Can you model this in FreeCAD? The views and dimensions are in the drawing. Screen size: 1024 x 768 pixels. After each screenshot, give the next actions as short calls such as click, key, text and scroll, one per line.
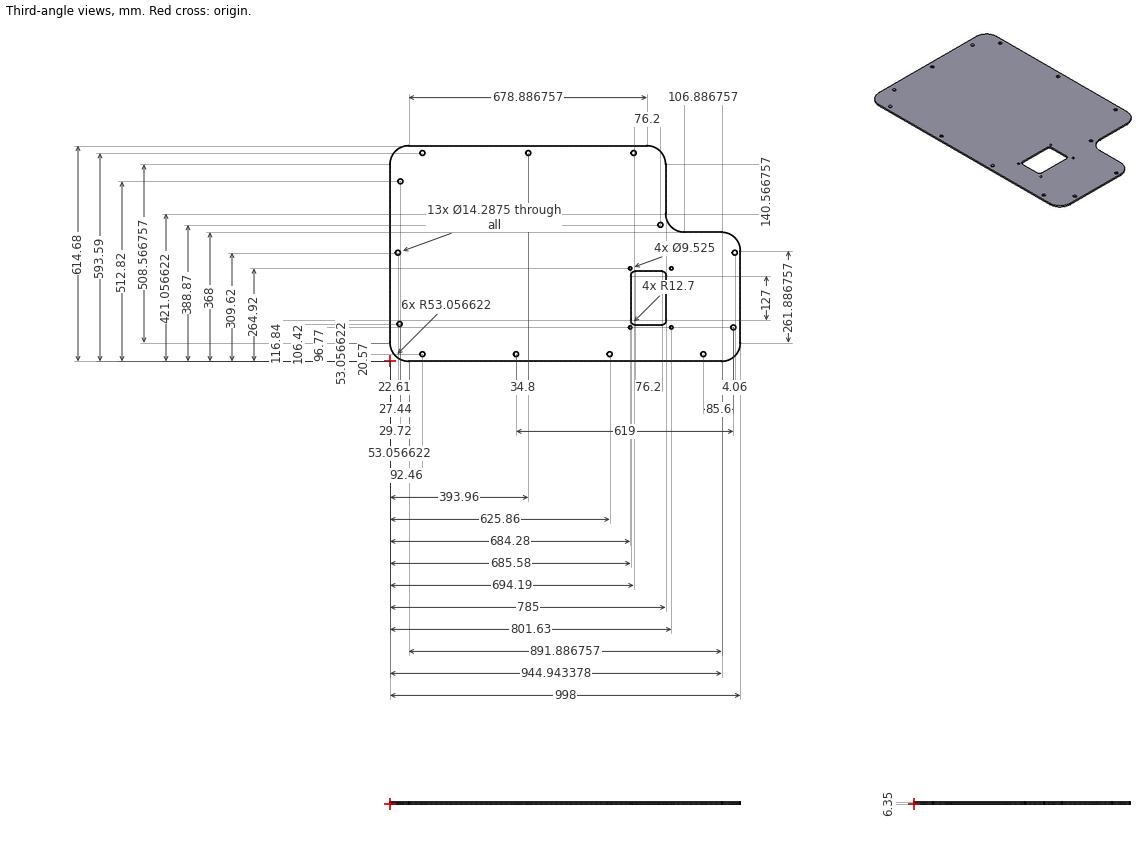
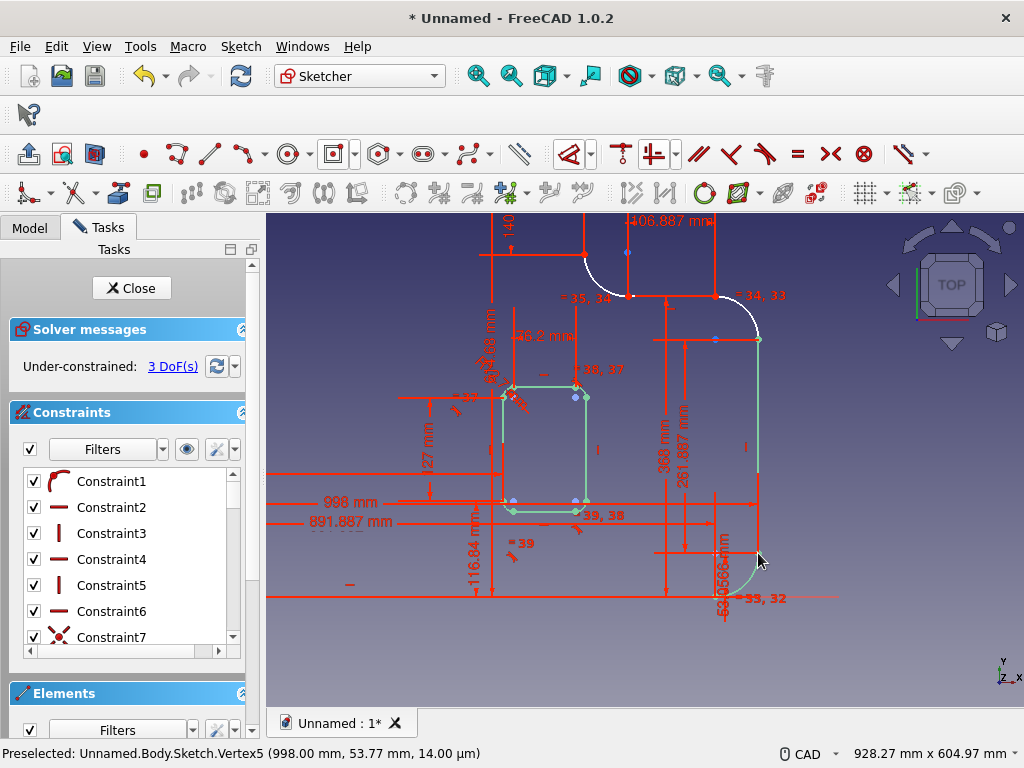
scroll(761, 553, down, 4)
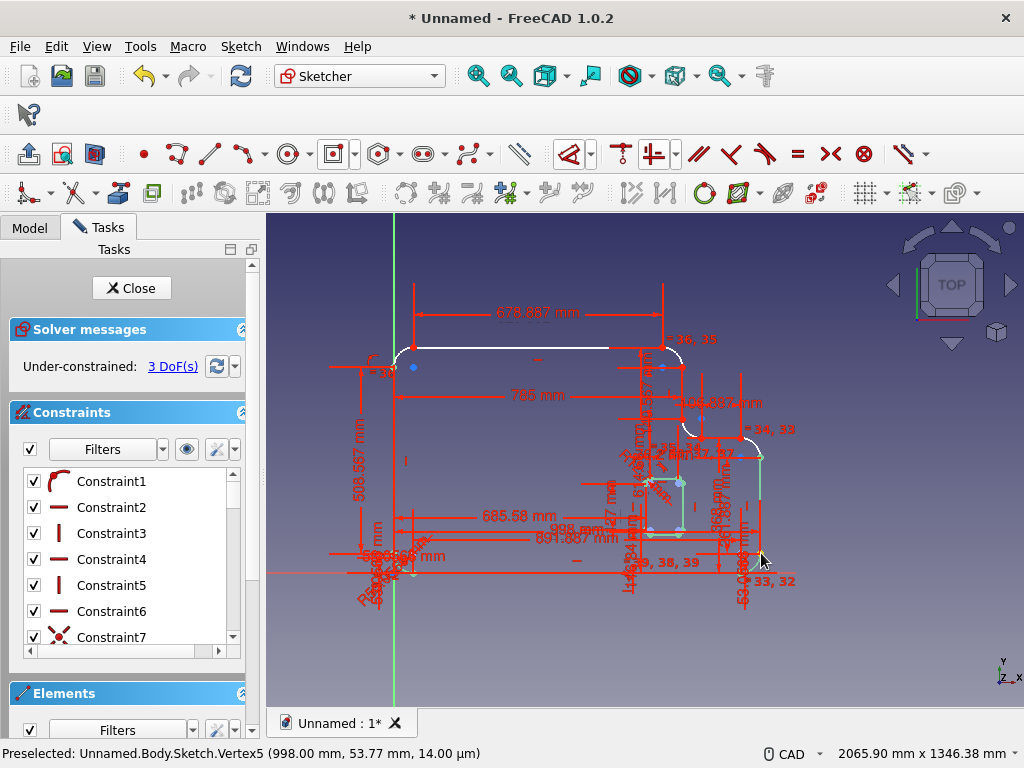
scroll(414, 348, up, 4)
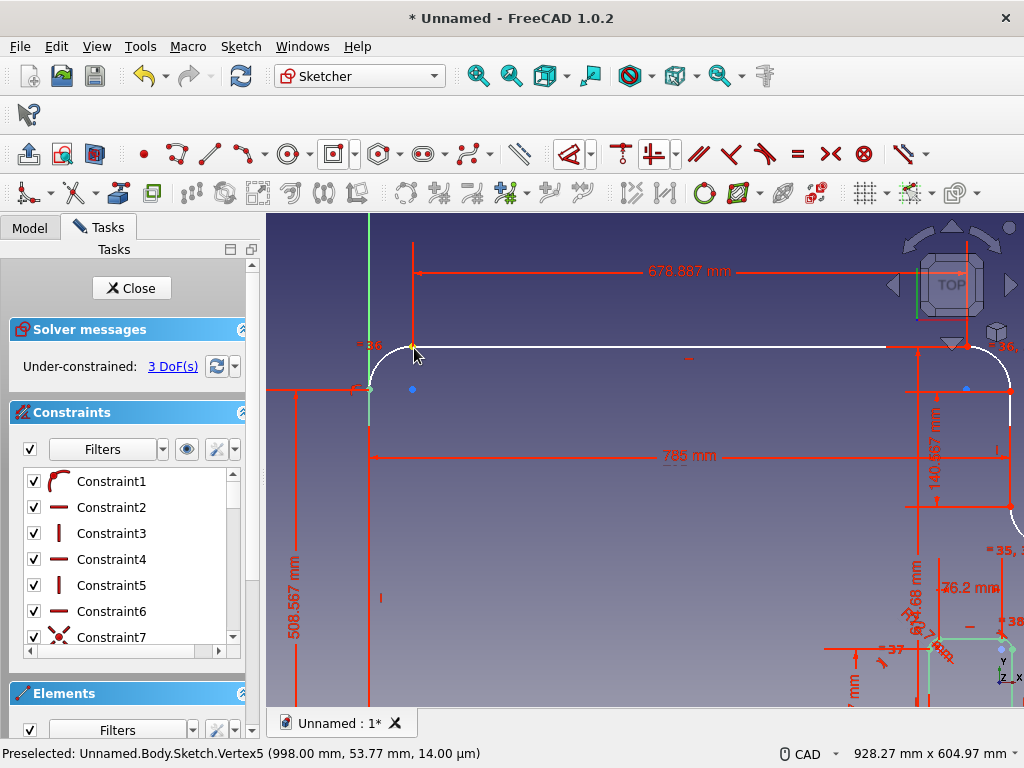
click(413, 347)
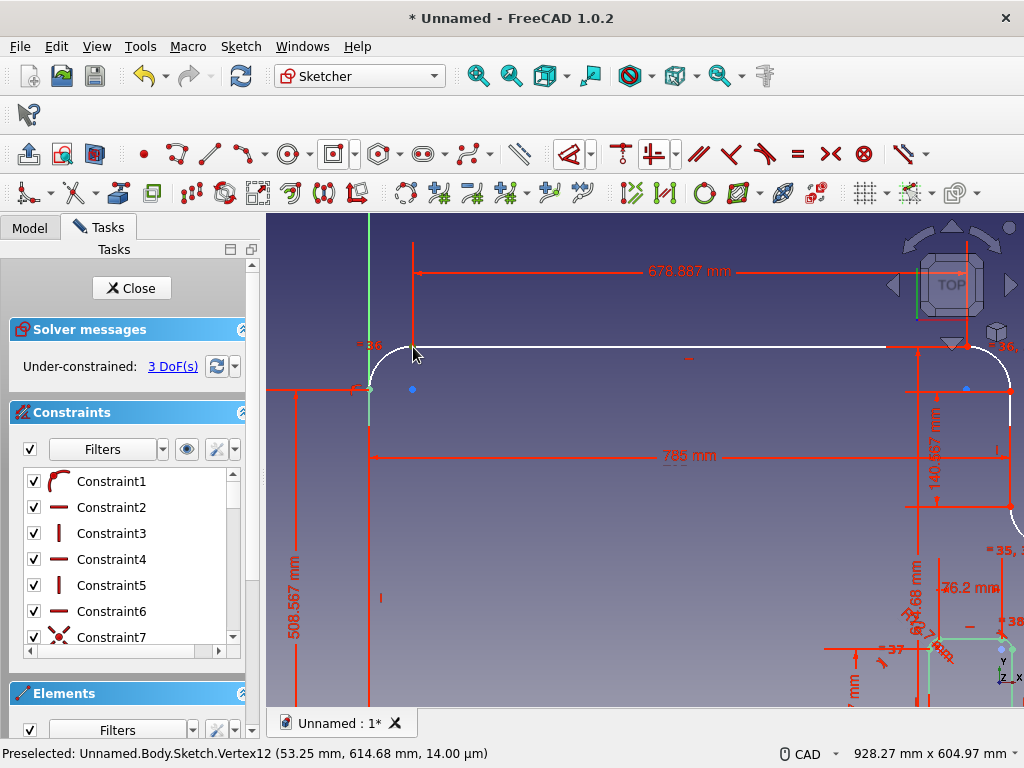
click(590, 154)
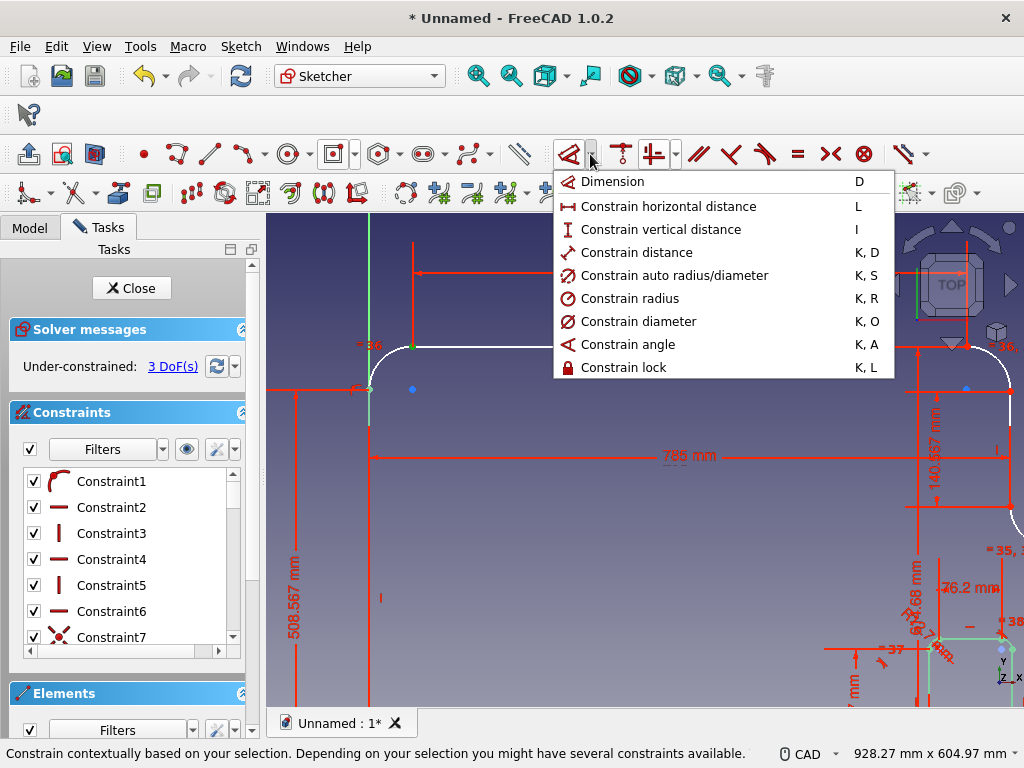
click(724, 206)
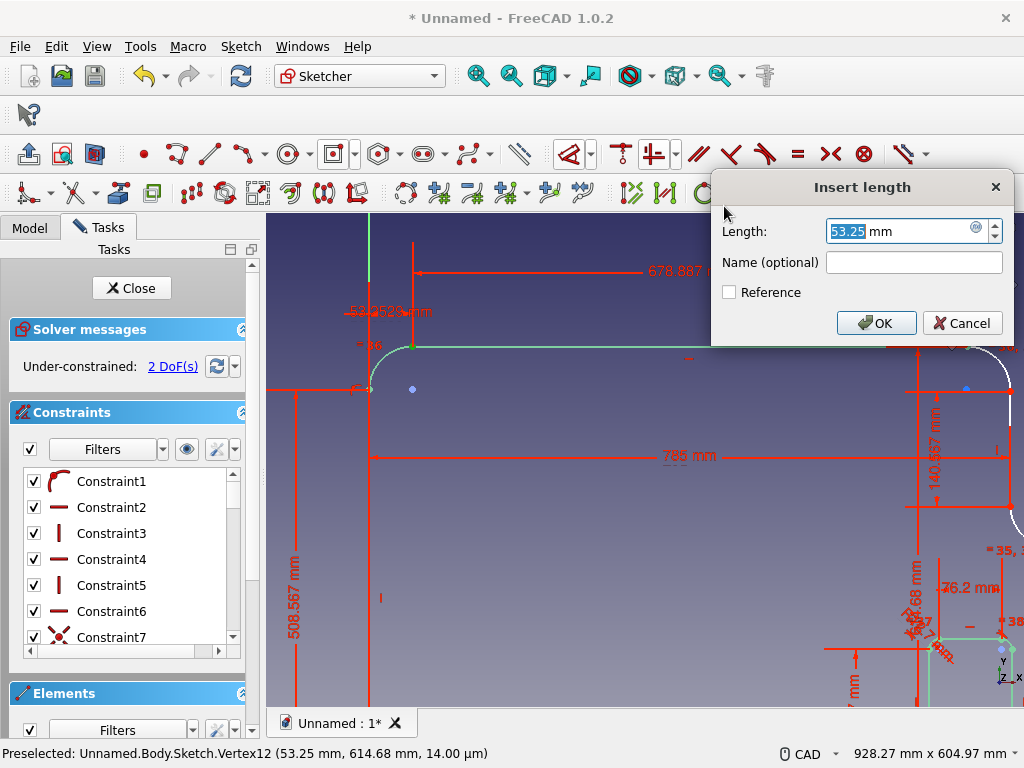
text(53.056622)
key(Return)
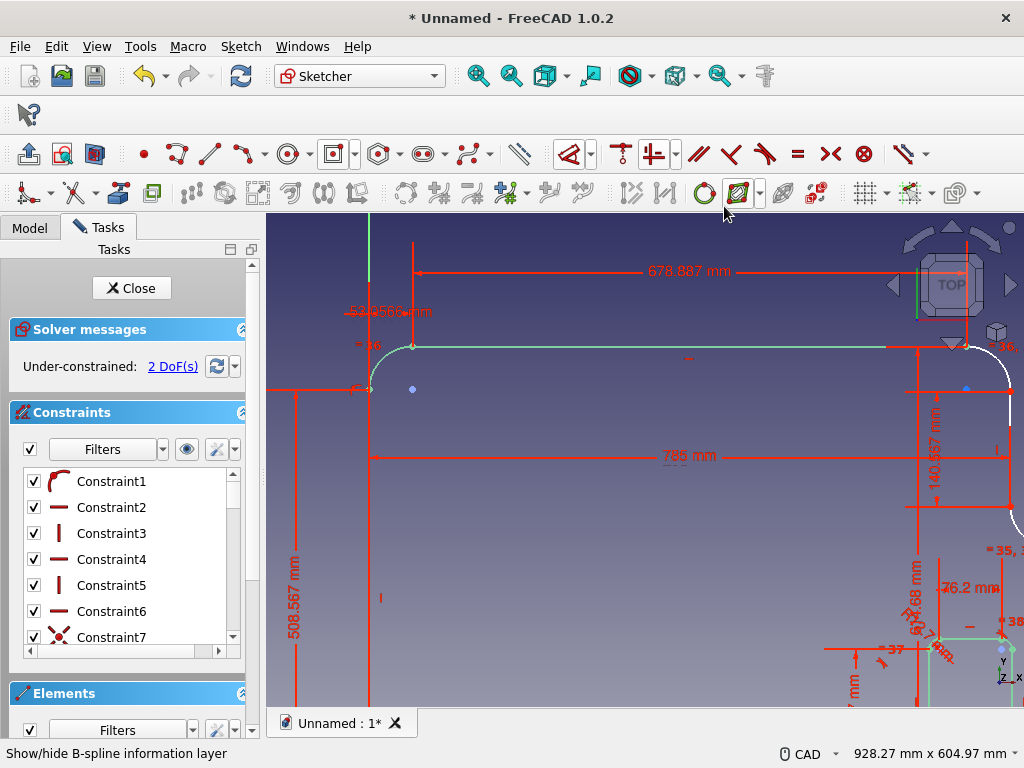
scroll(413, 348, down, 4)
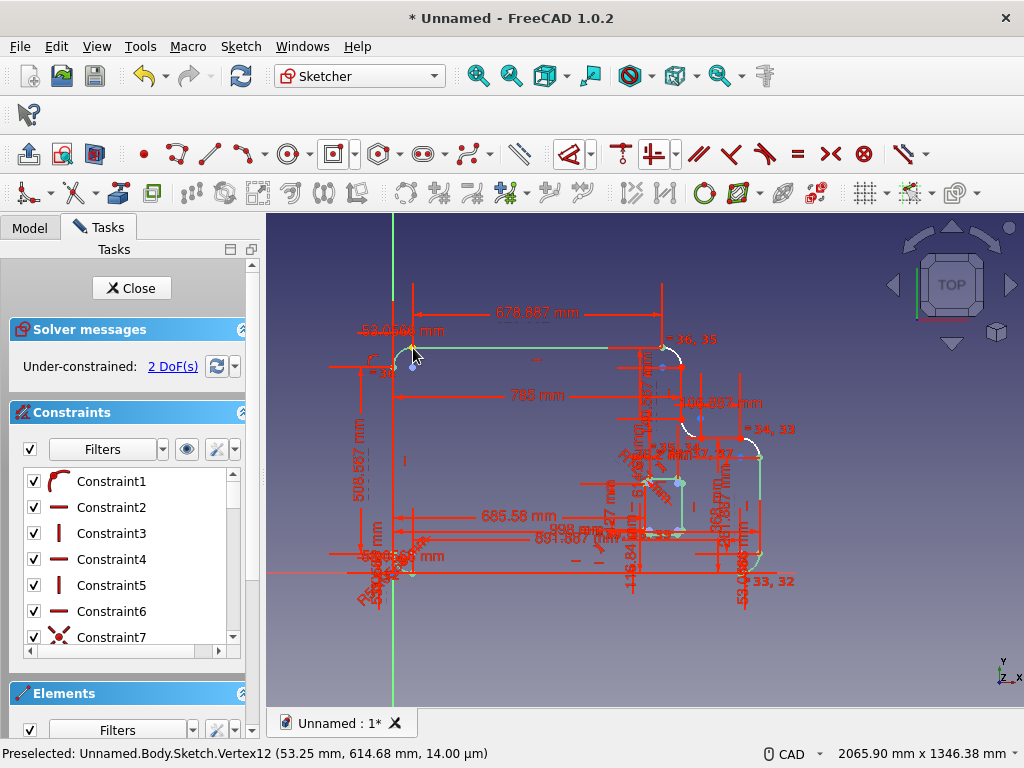
click(740, 438)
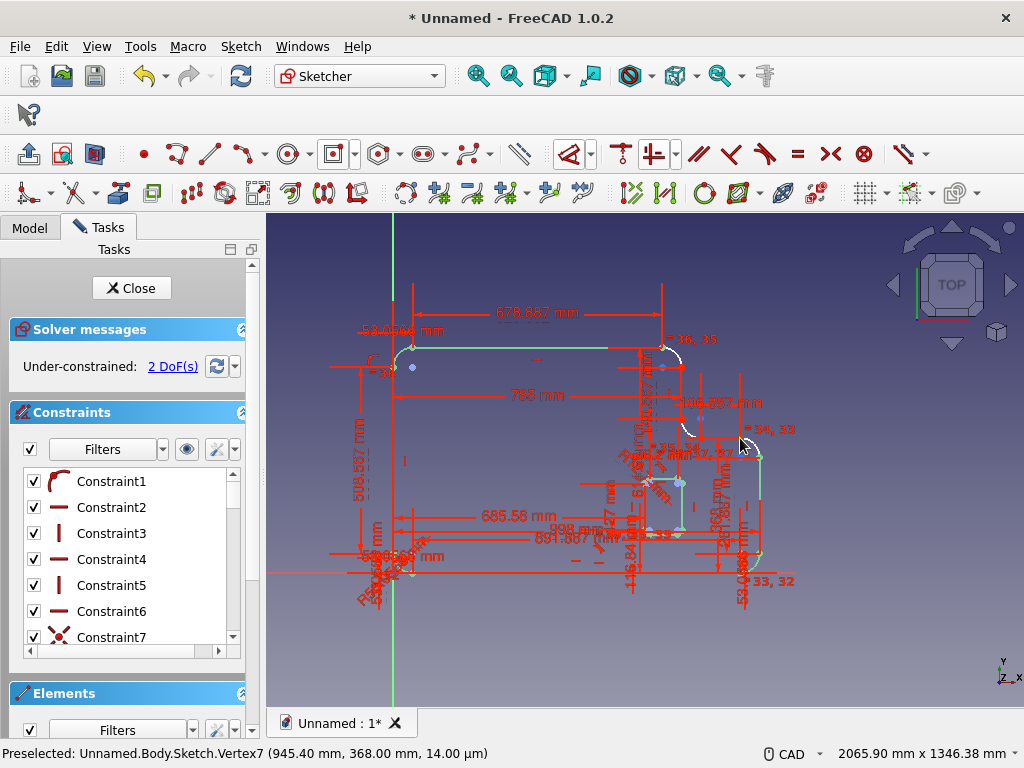
click(590, 154)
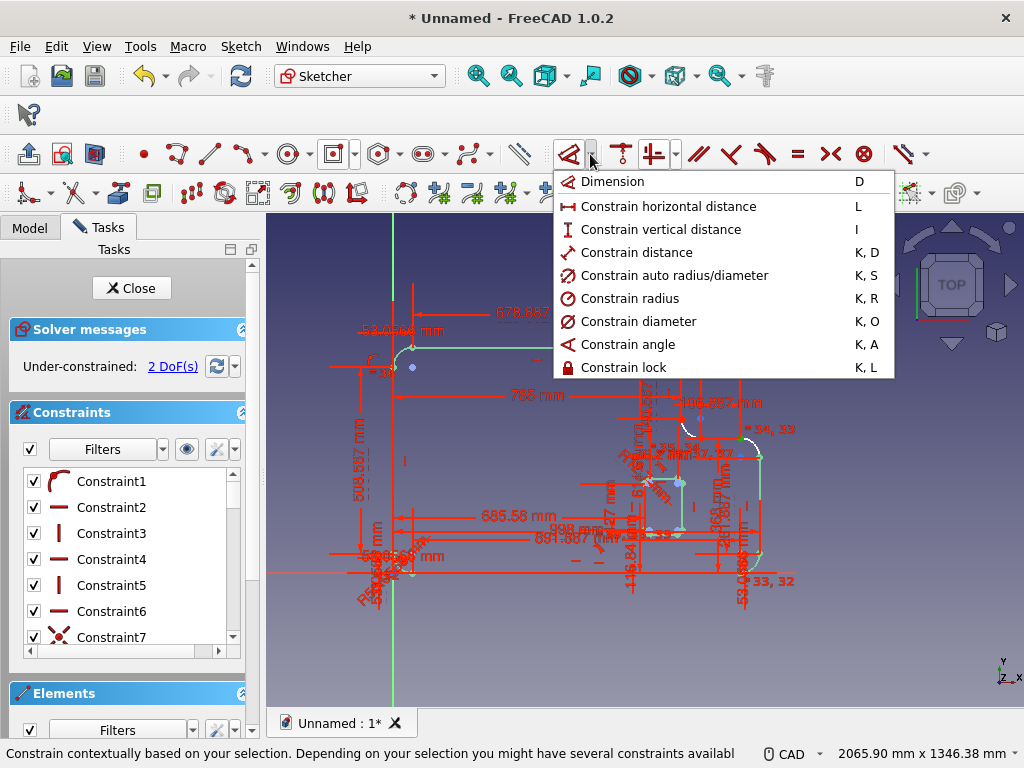
click(724, 206)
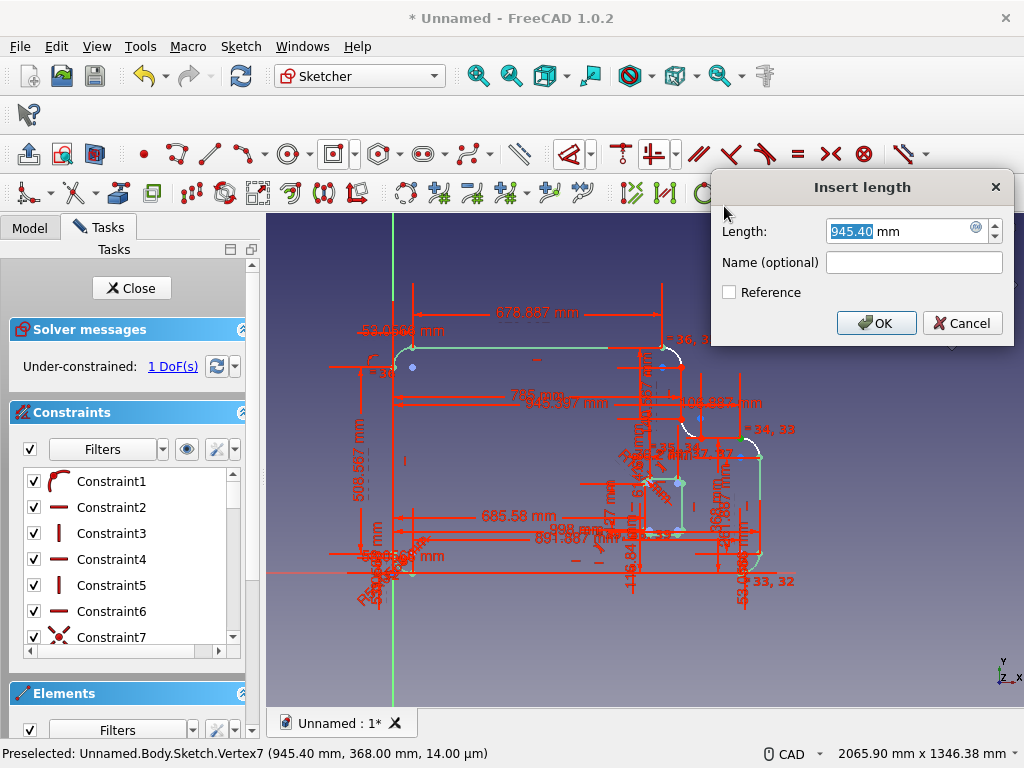
text(944.943378)
key(Return)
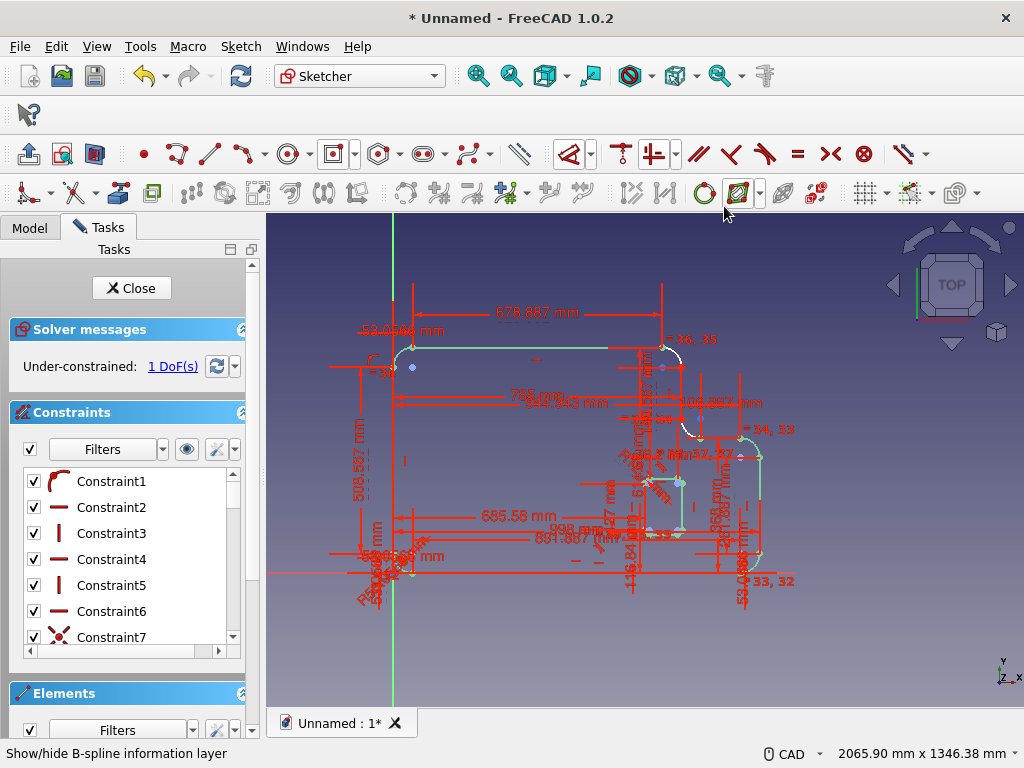
click(681, 419)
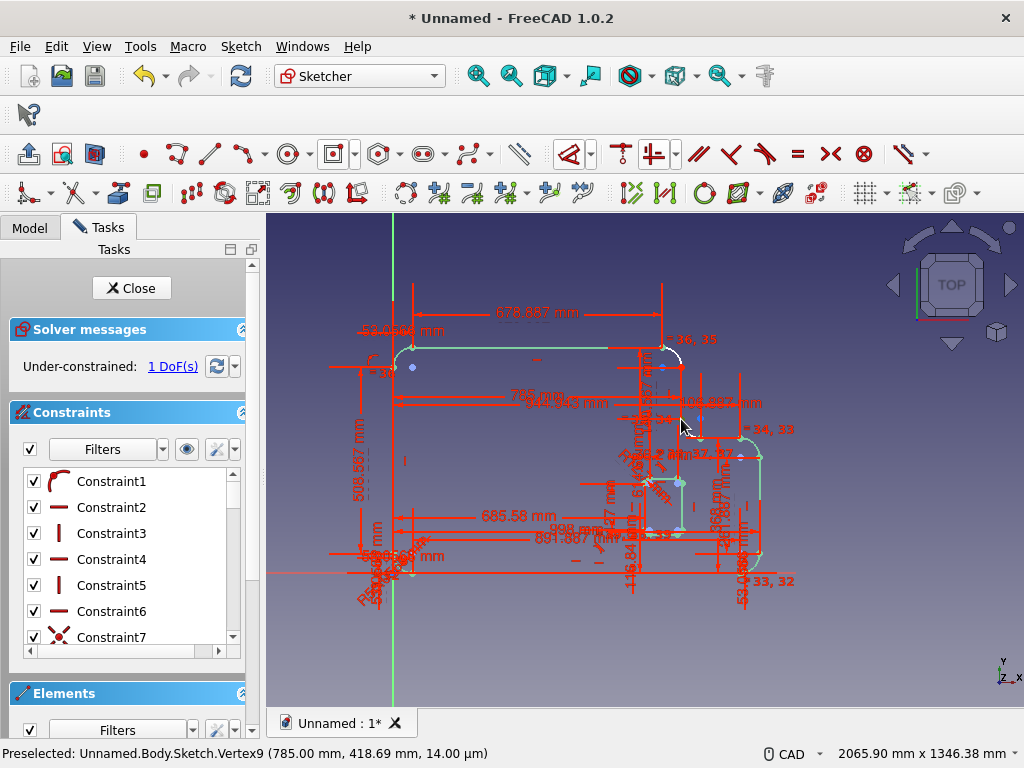
key(i)